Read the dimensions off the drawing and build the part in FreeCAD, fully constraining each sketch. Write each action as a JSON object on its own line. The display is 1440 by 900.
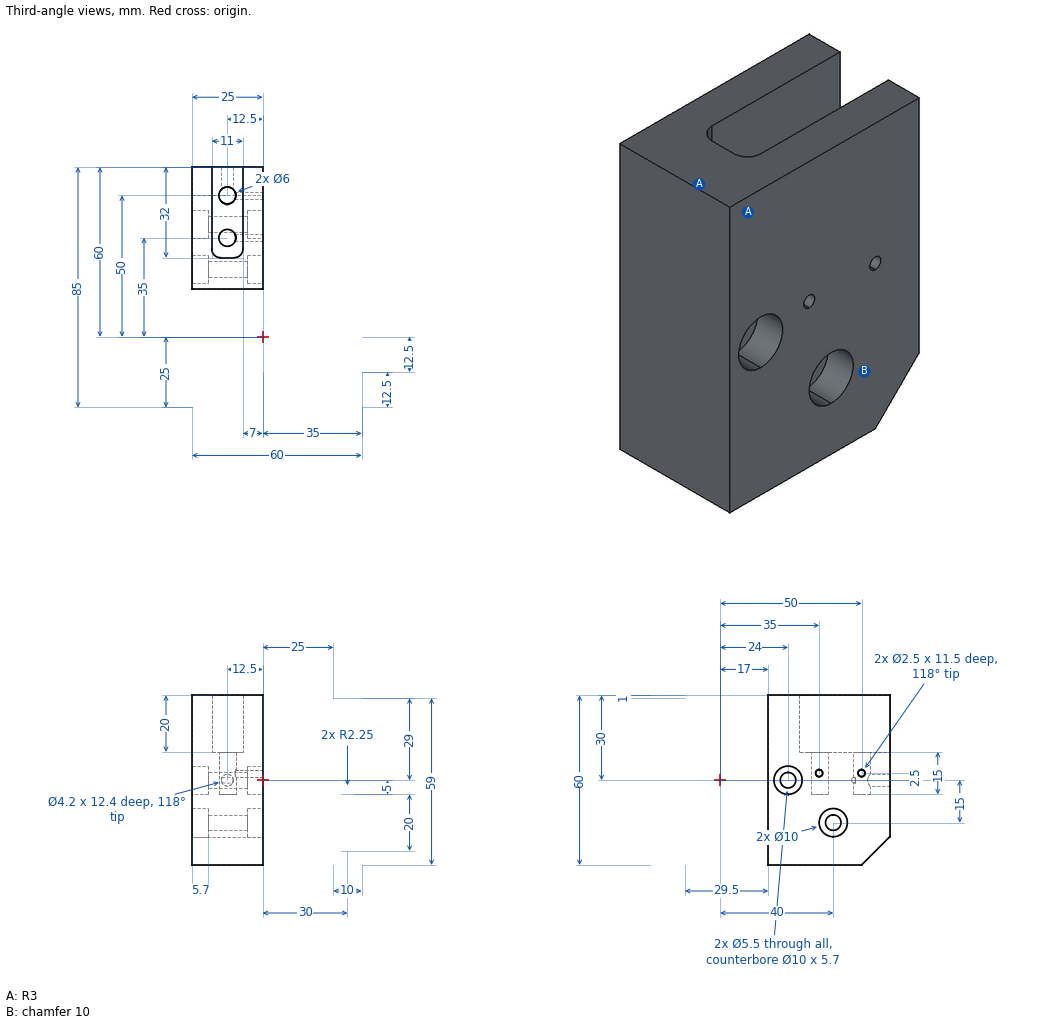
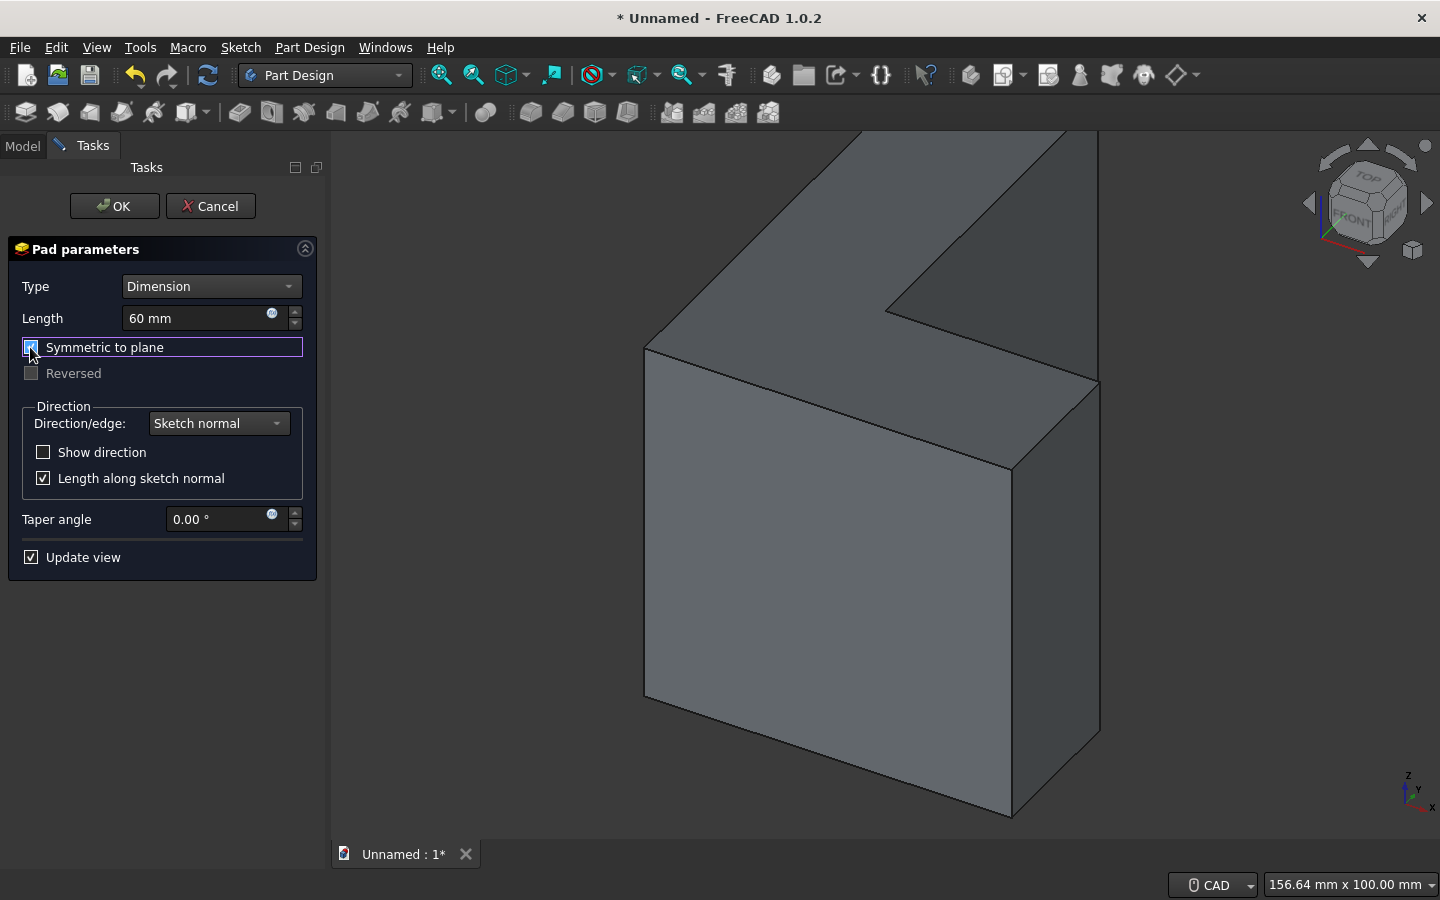
{"action": "left_click", "coordinate": [115, 206]}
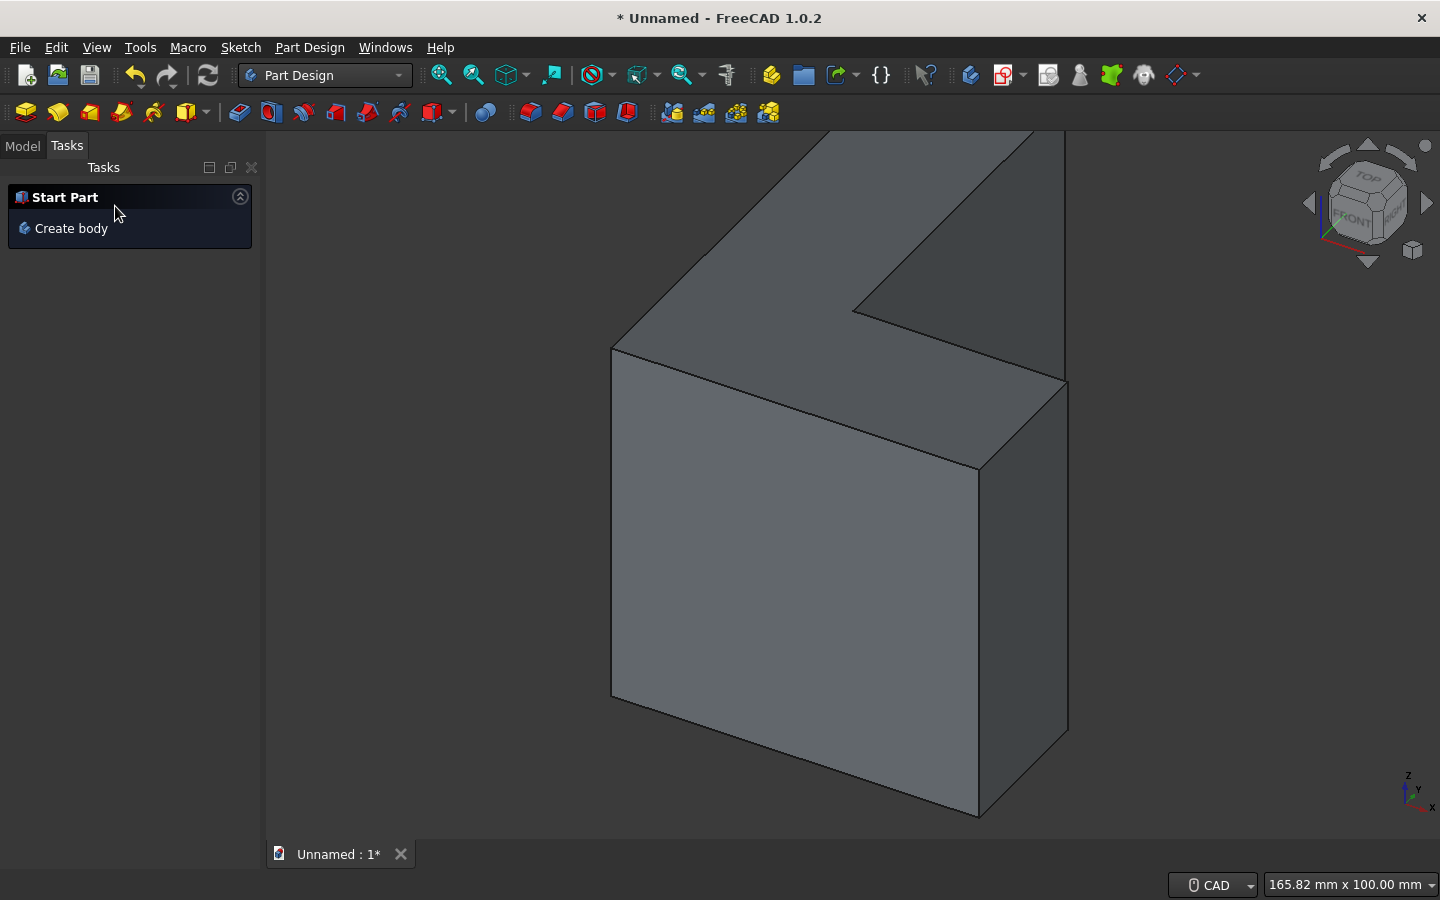
{"action": "left_click", "coordinate": [442, 76]}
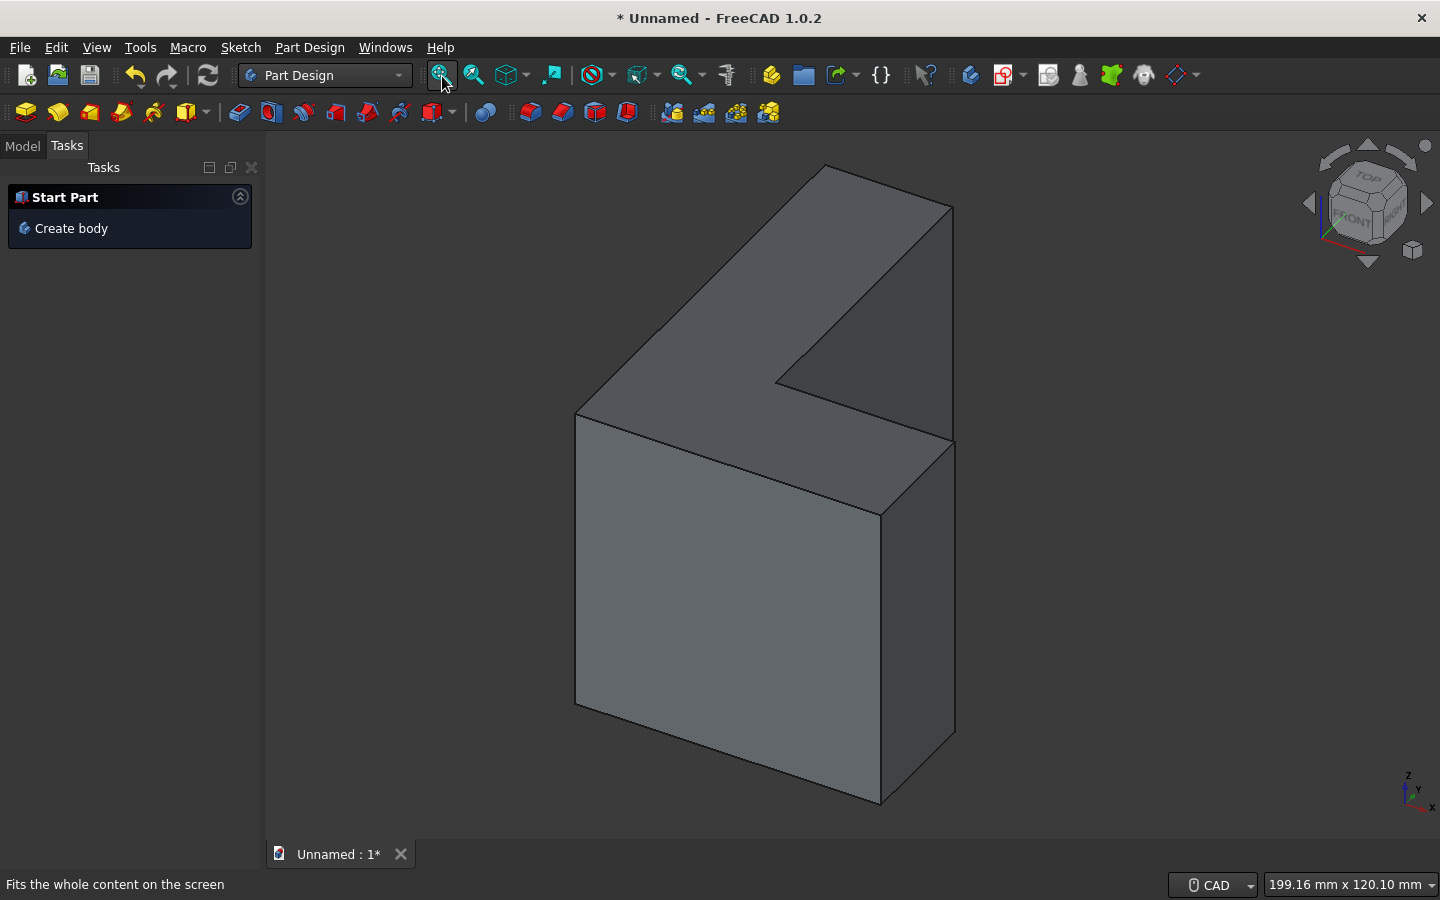
{"action": "left_click", "coordinate": [694, 381]}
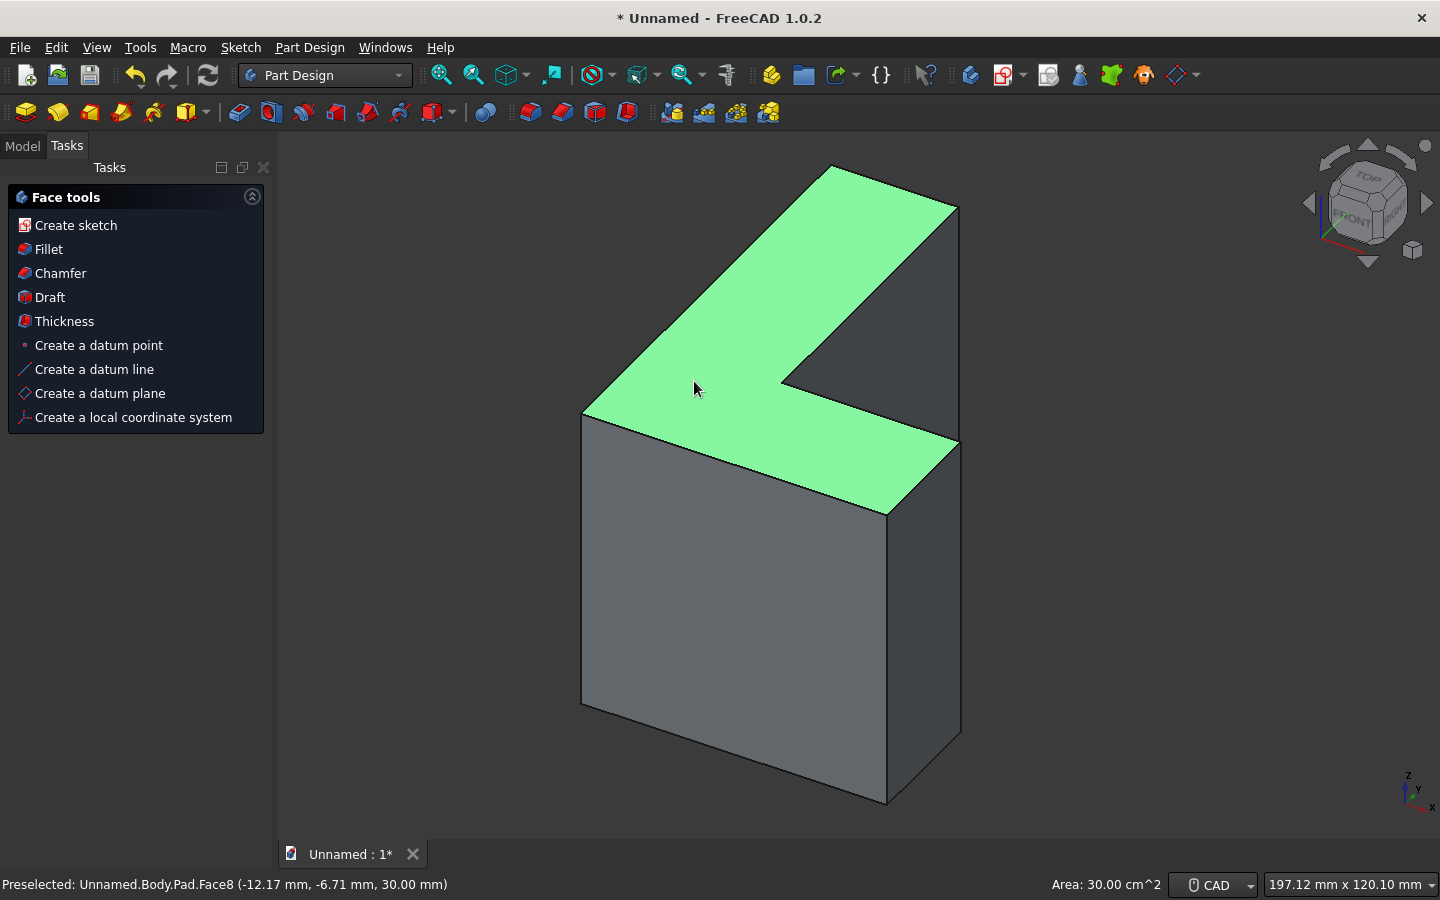
{"action": "left_click", "coordinate": [1004, 76]}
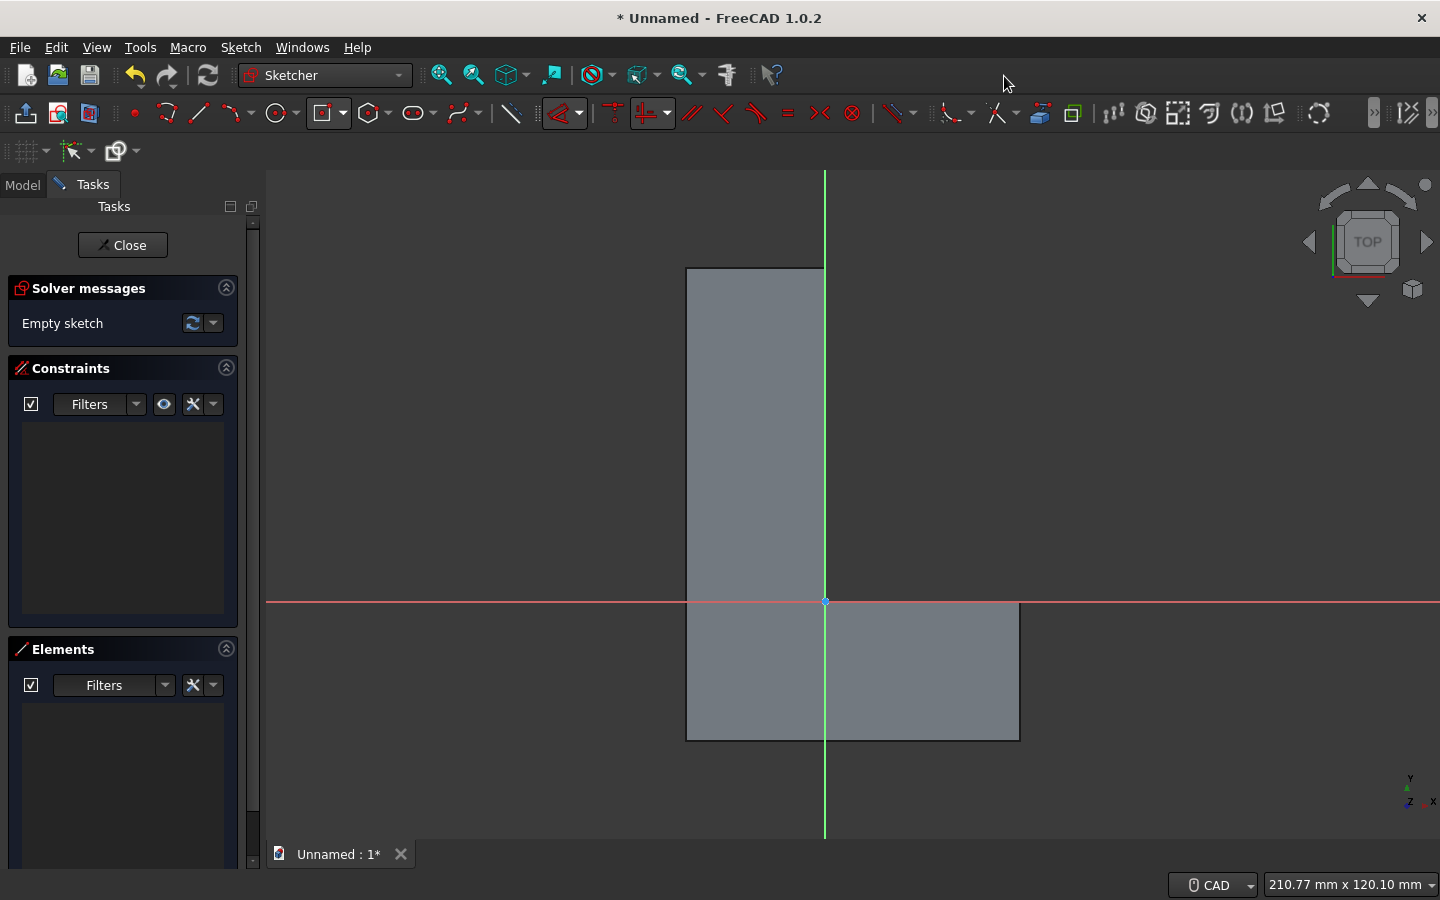
{"action": "scroll", "coordinate": [909, 808], "scroll_direction": "up", "scroll_amount": 4}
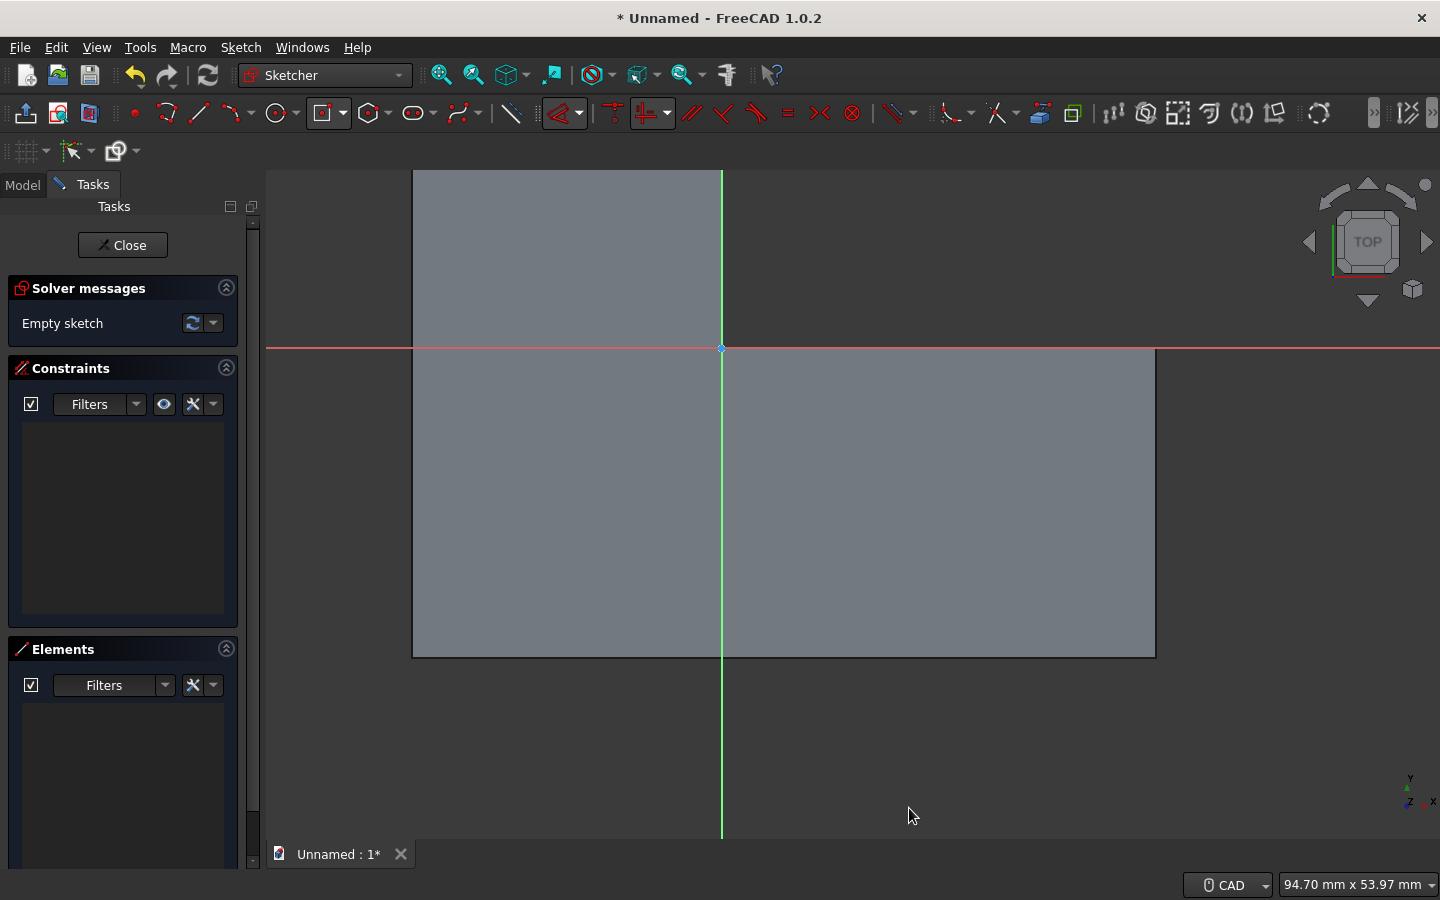
{"action": "key", "text": "g r"}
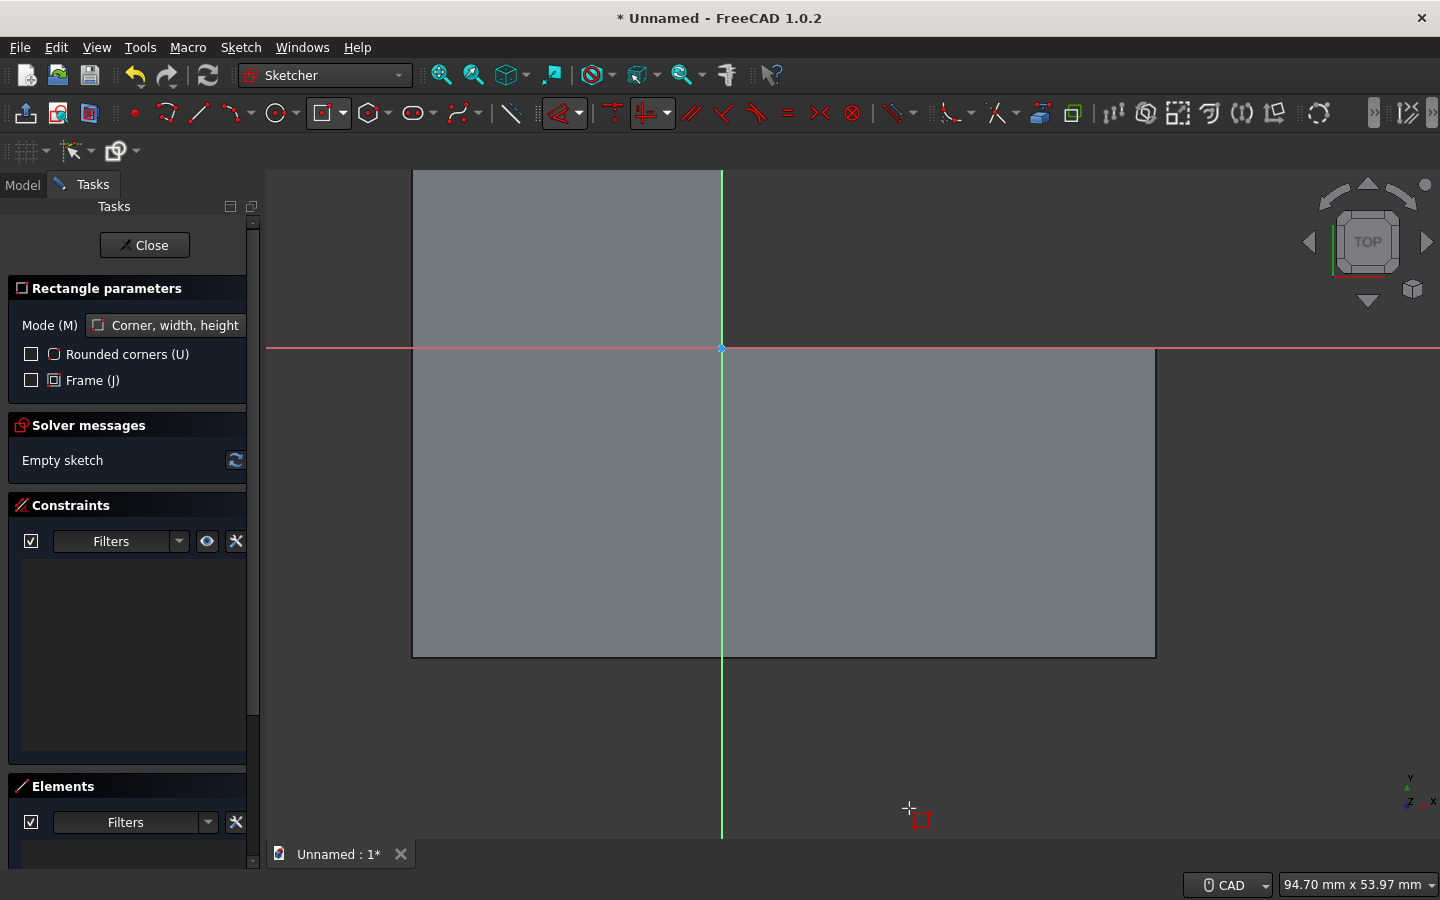
{"action": "left_click", "coordinate": [412, 503]}
{"action": "mouse_move", "coordinate": [1156, 658]}